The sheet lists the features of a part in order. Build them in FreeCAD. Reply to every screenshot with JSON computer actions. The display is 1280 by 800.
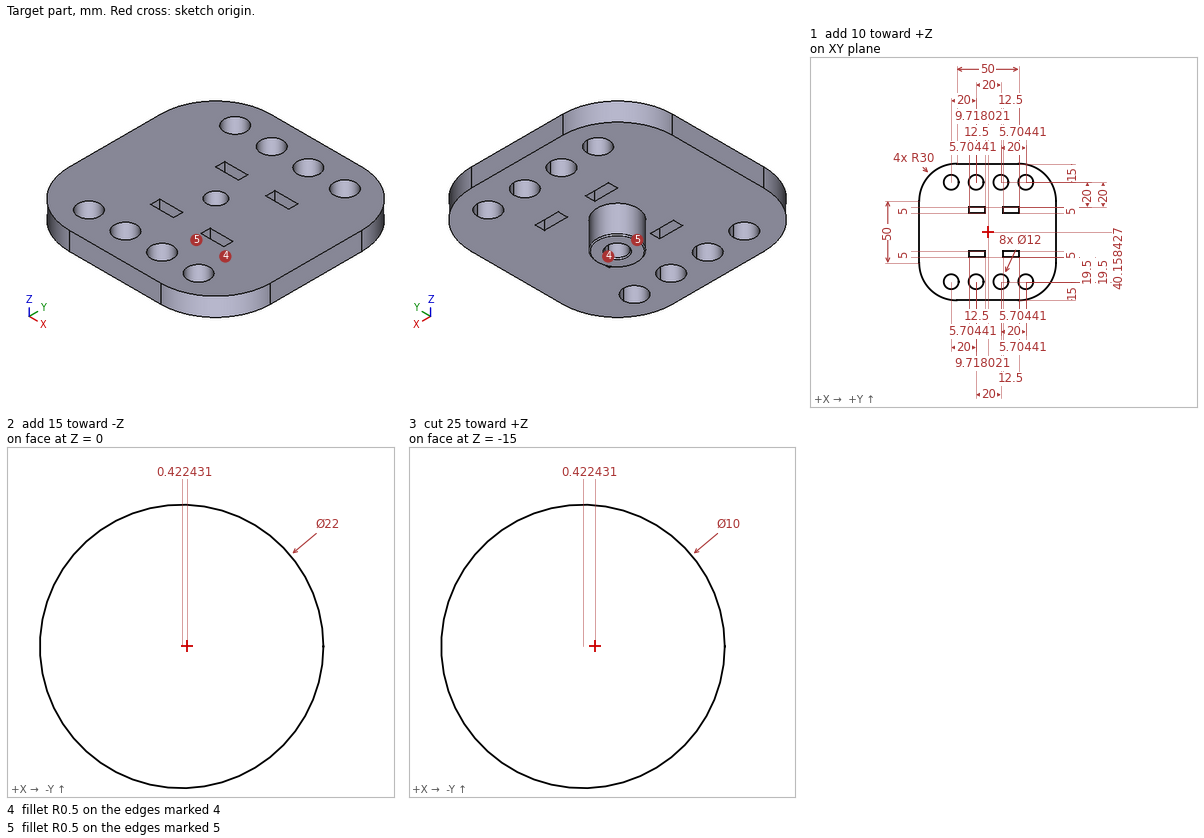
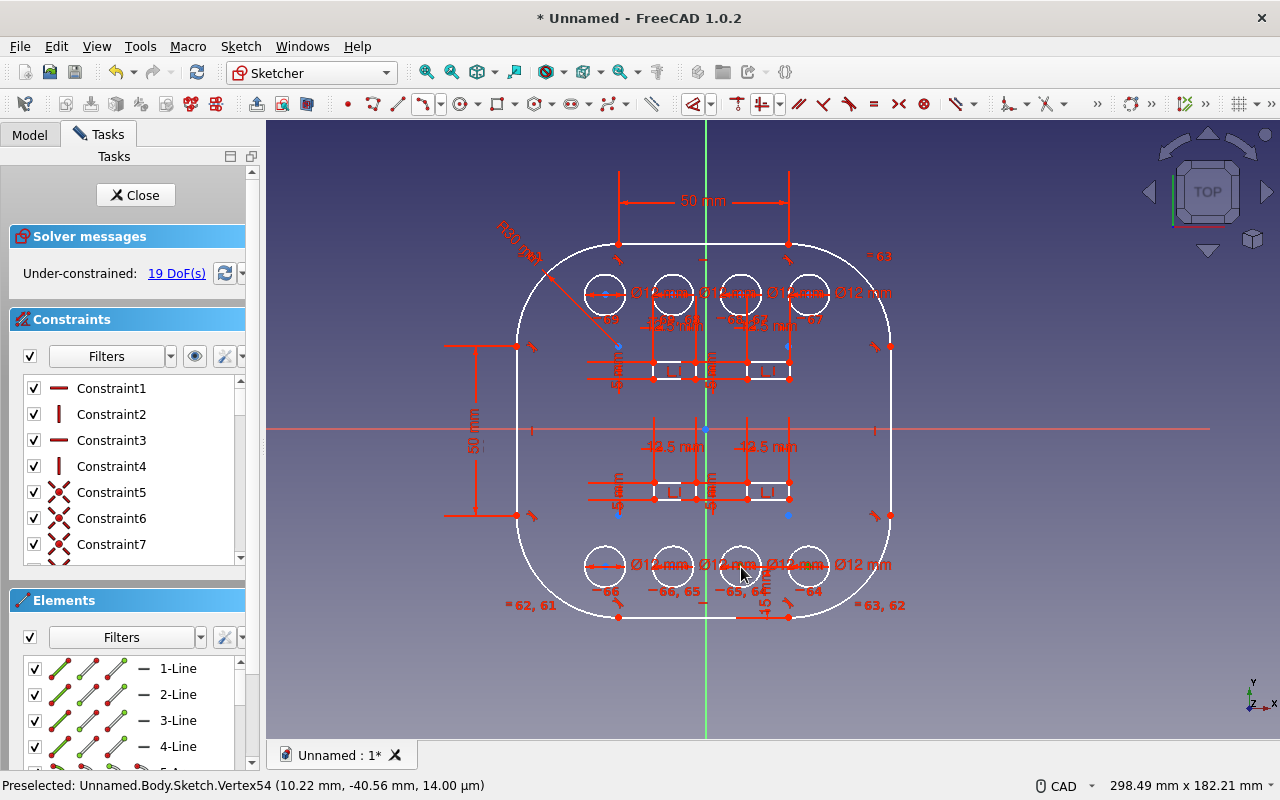
{"action": "key", "text": "l"}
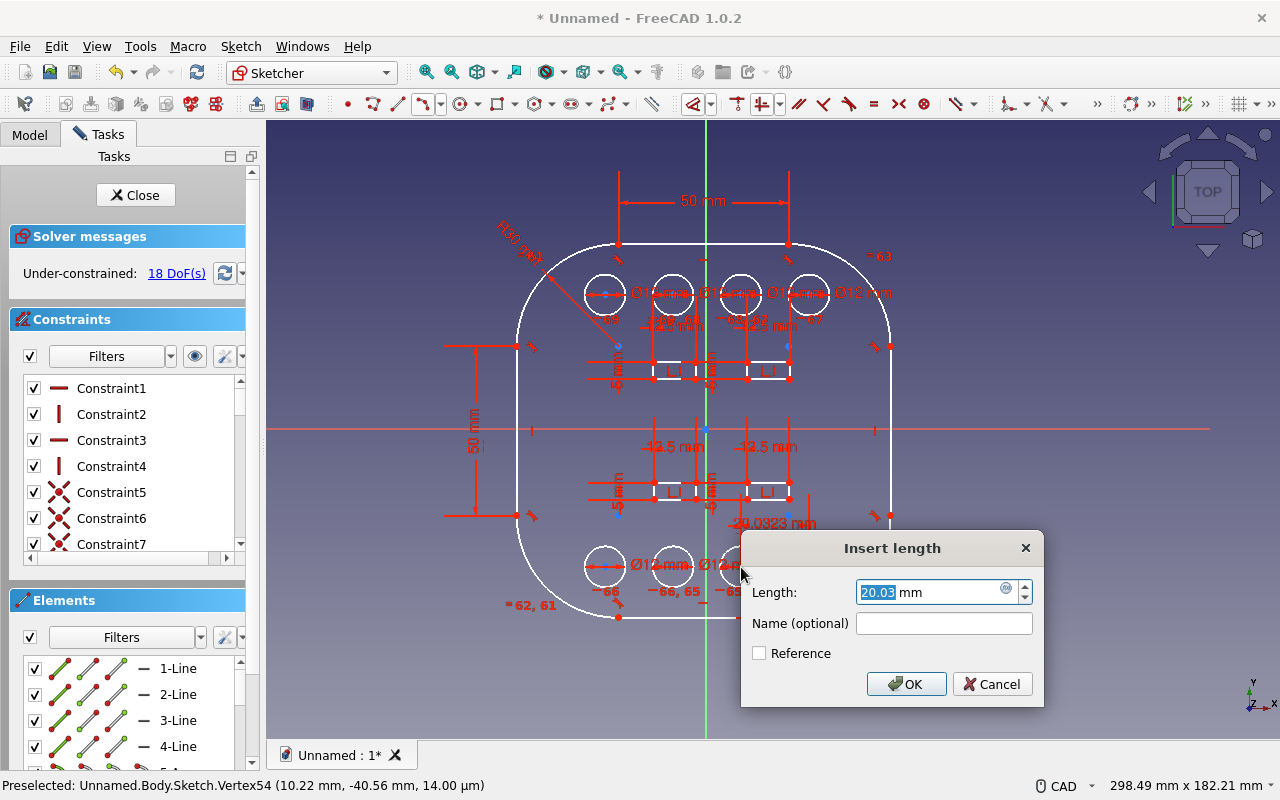
{"action": "type", "text": "20"}
{"action": "key", "text": "Return"}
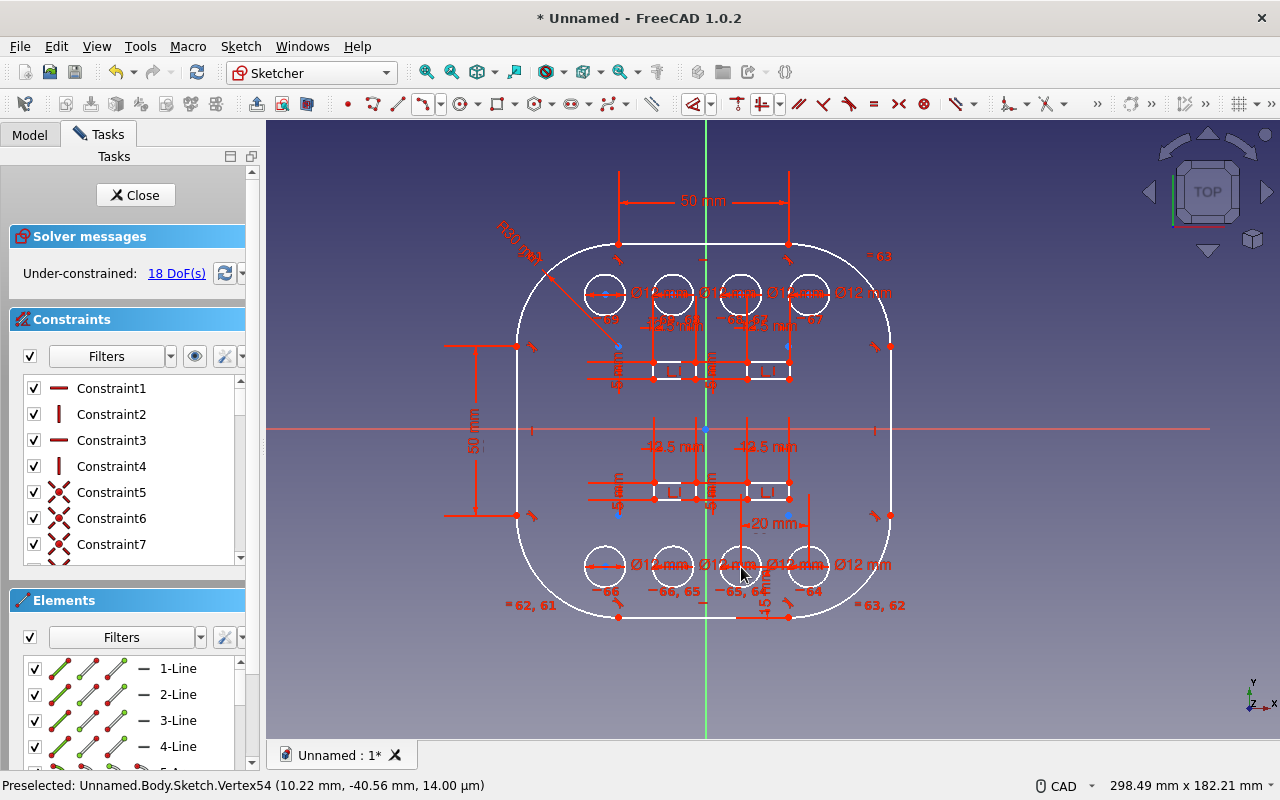
{"action": "left_click", "coordinate": [741, 567]}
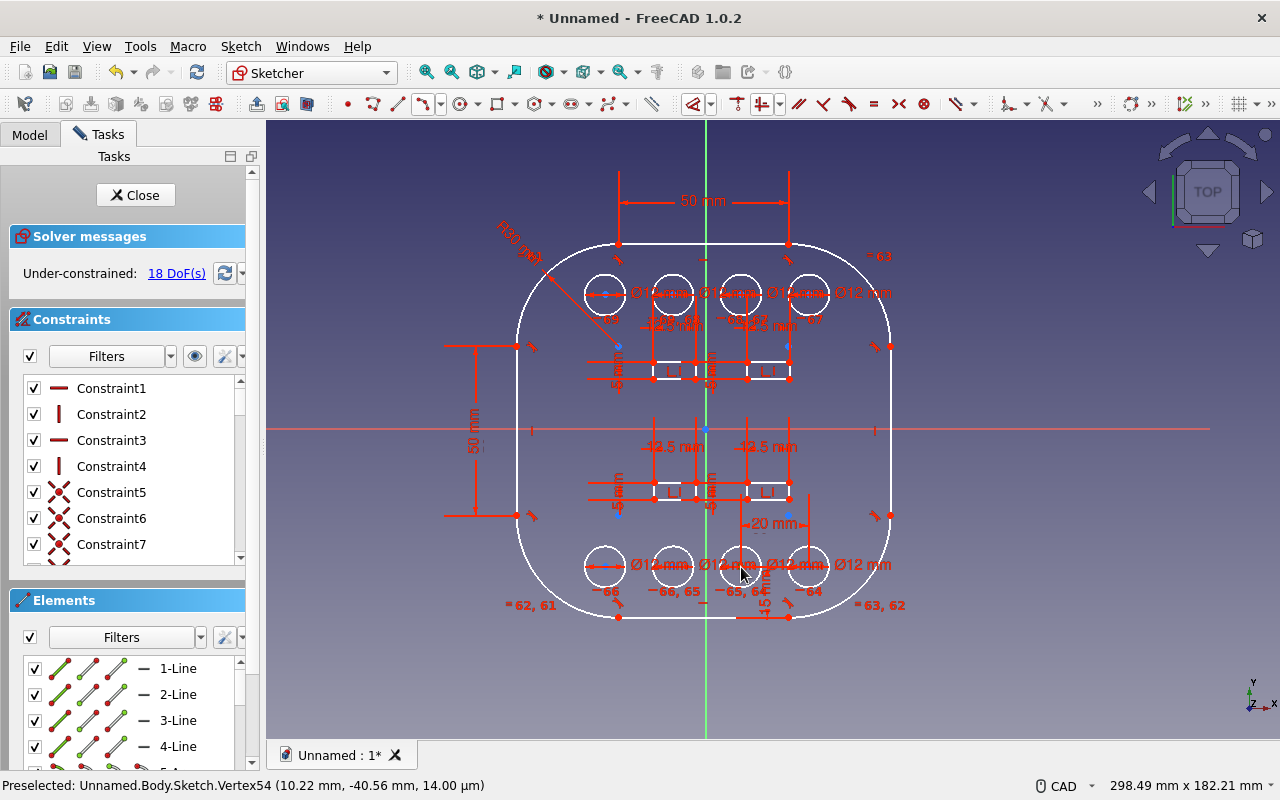
{"action": "left_click", "coordinate": [673, 567]}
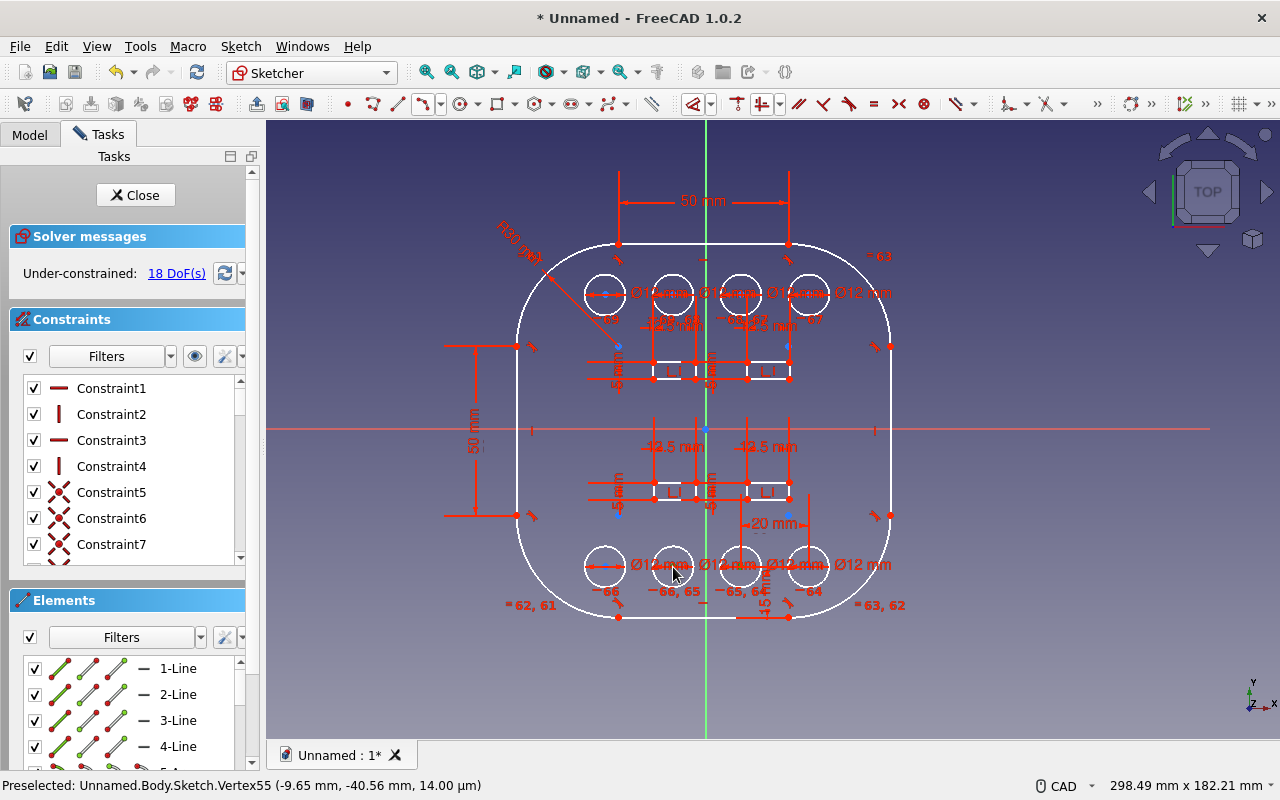
{"action": "left_click", "coordinate": [710, 104]}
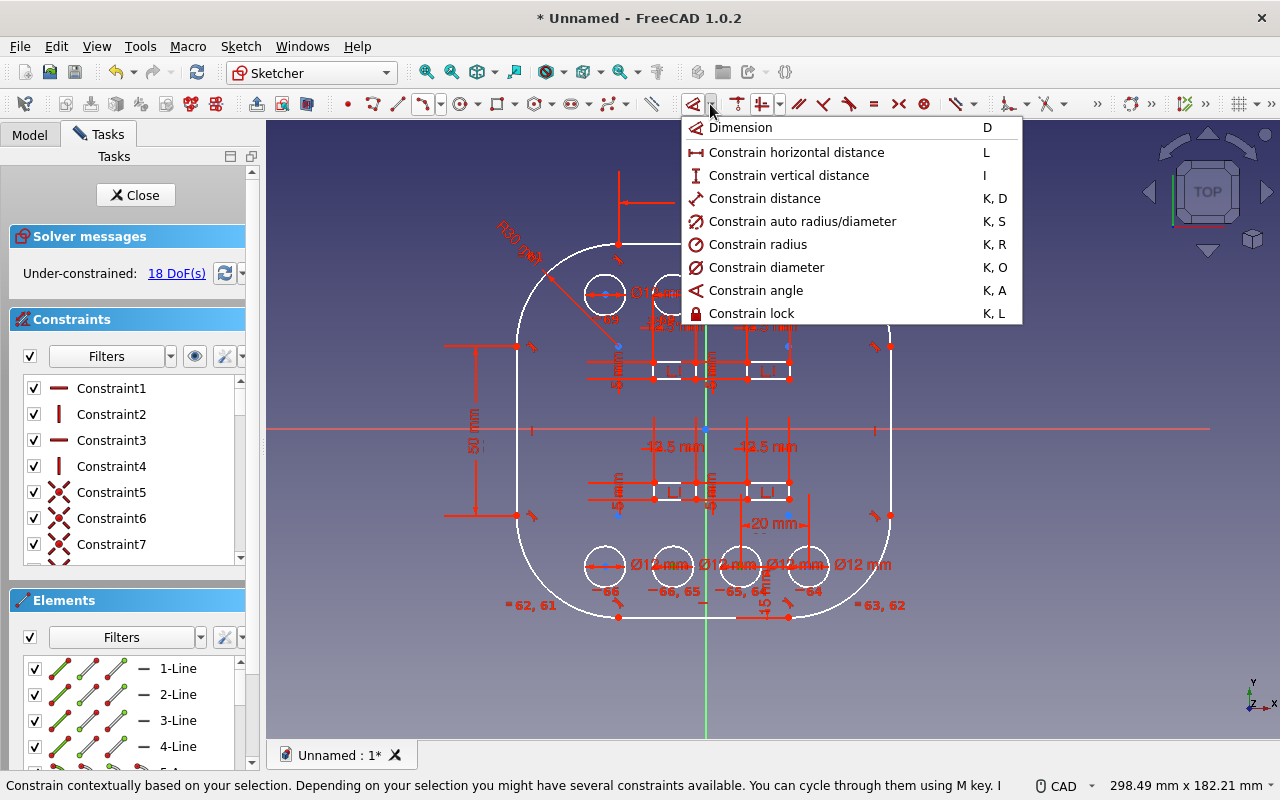
{"action": "left_click", "coordinate": [852, 152]}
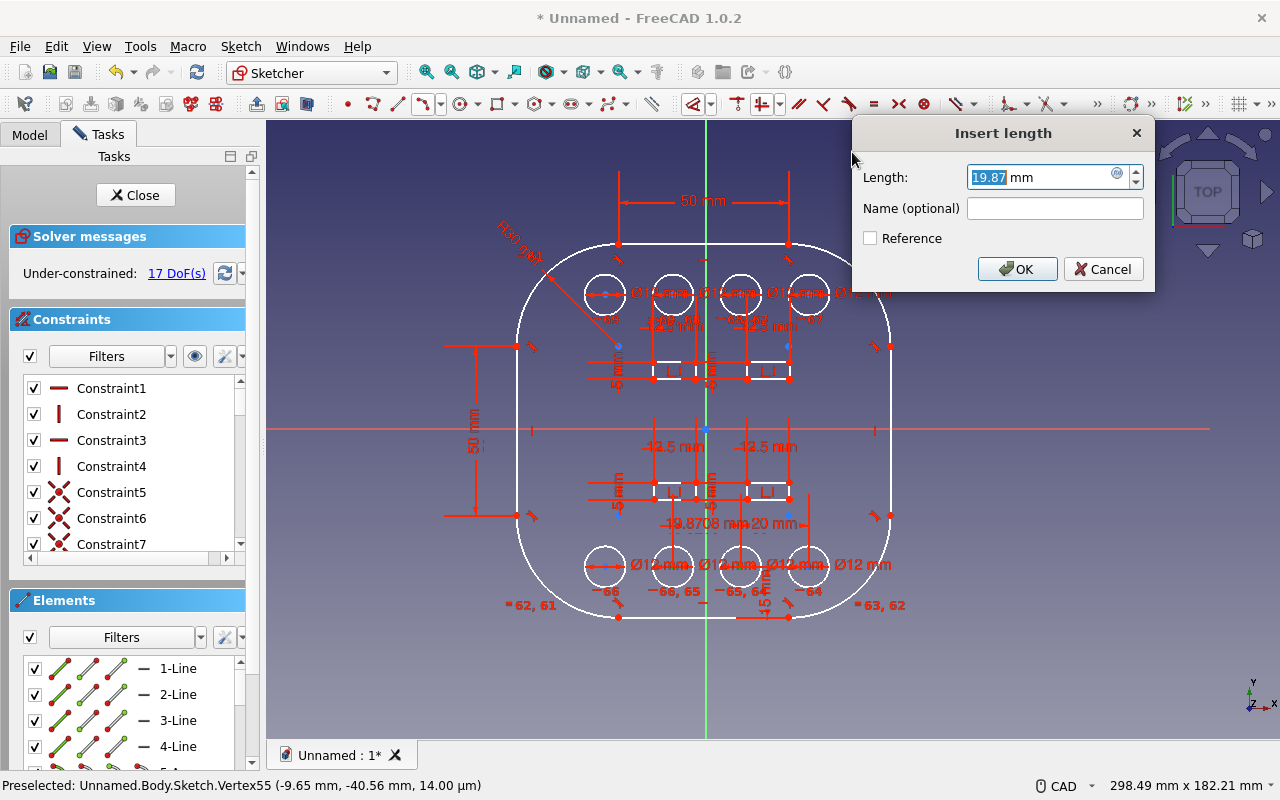
{"action": "type", "text": "20"}
{"action": "key", "text": "Return"}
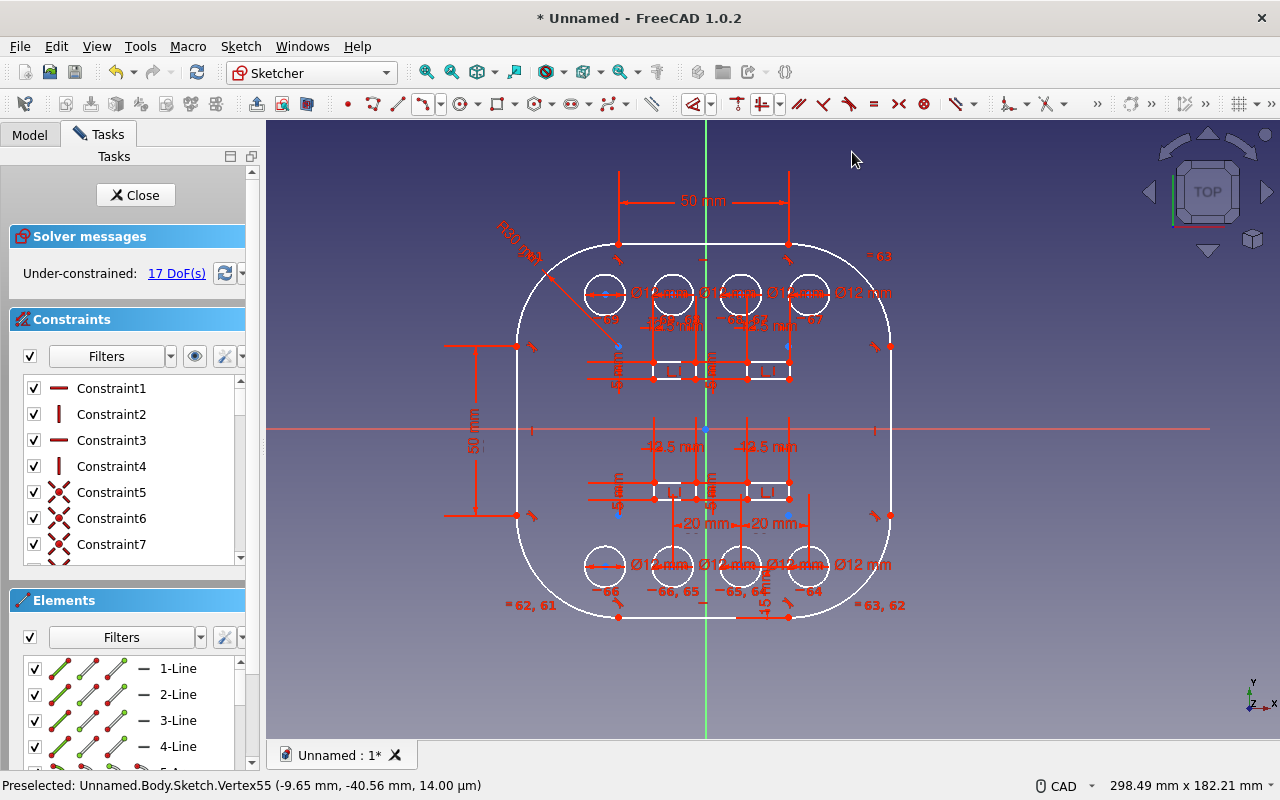
{"action": "left_click", "coordinate": [673, 567]}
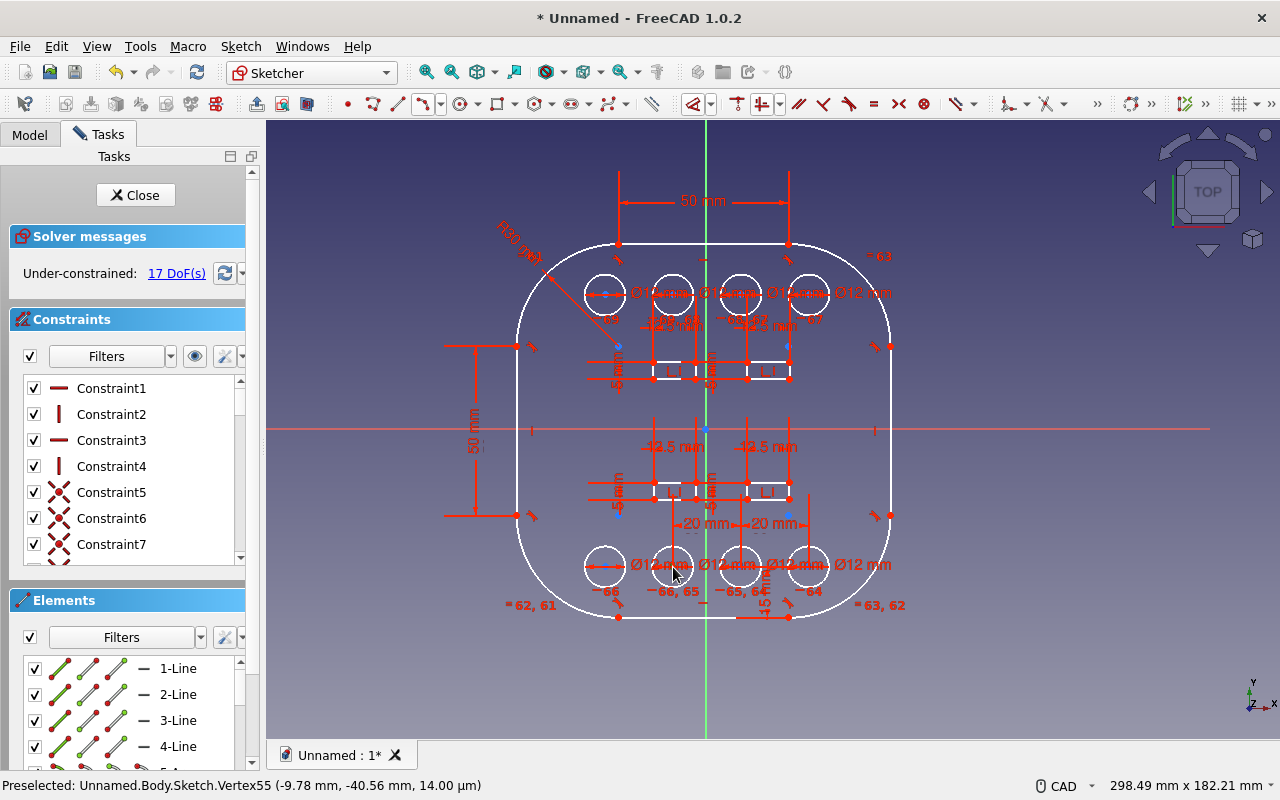
{"action": "left_click", "coordinate": [605, 567]}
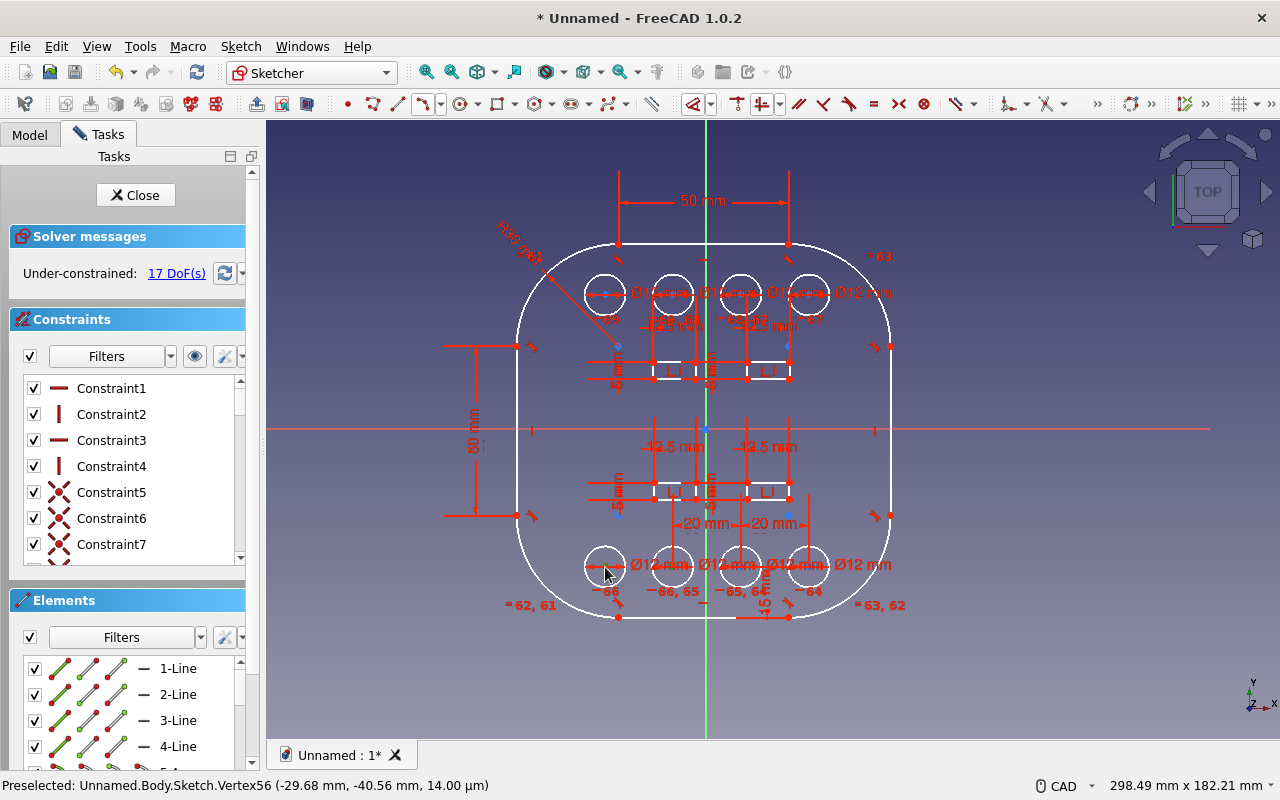
{"action": "left_click", "coordinate": [710, 104]}